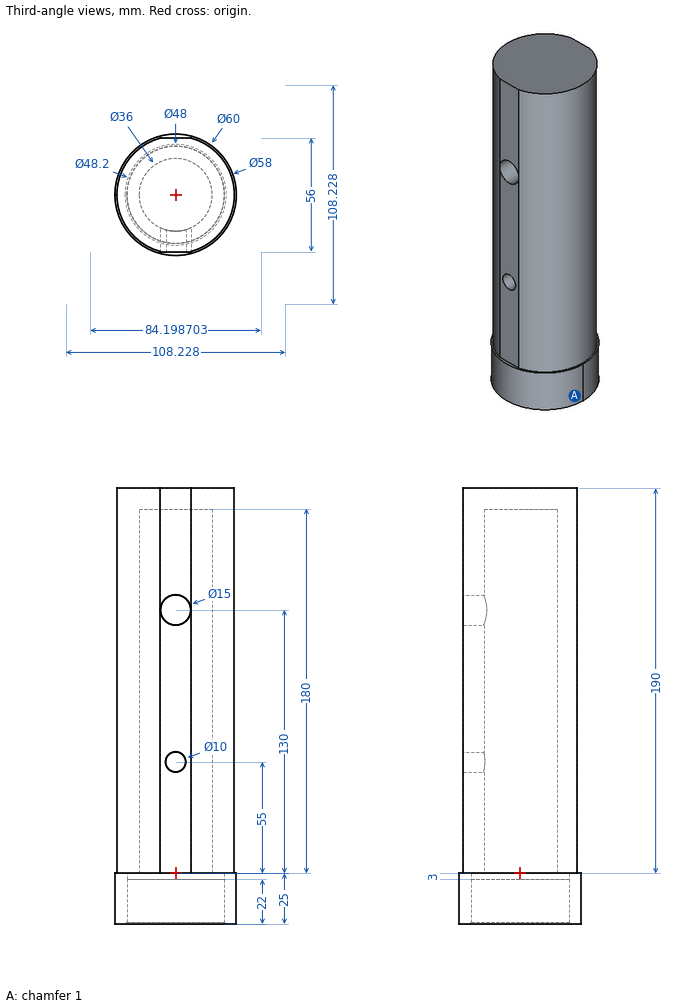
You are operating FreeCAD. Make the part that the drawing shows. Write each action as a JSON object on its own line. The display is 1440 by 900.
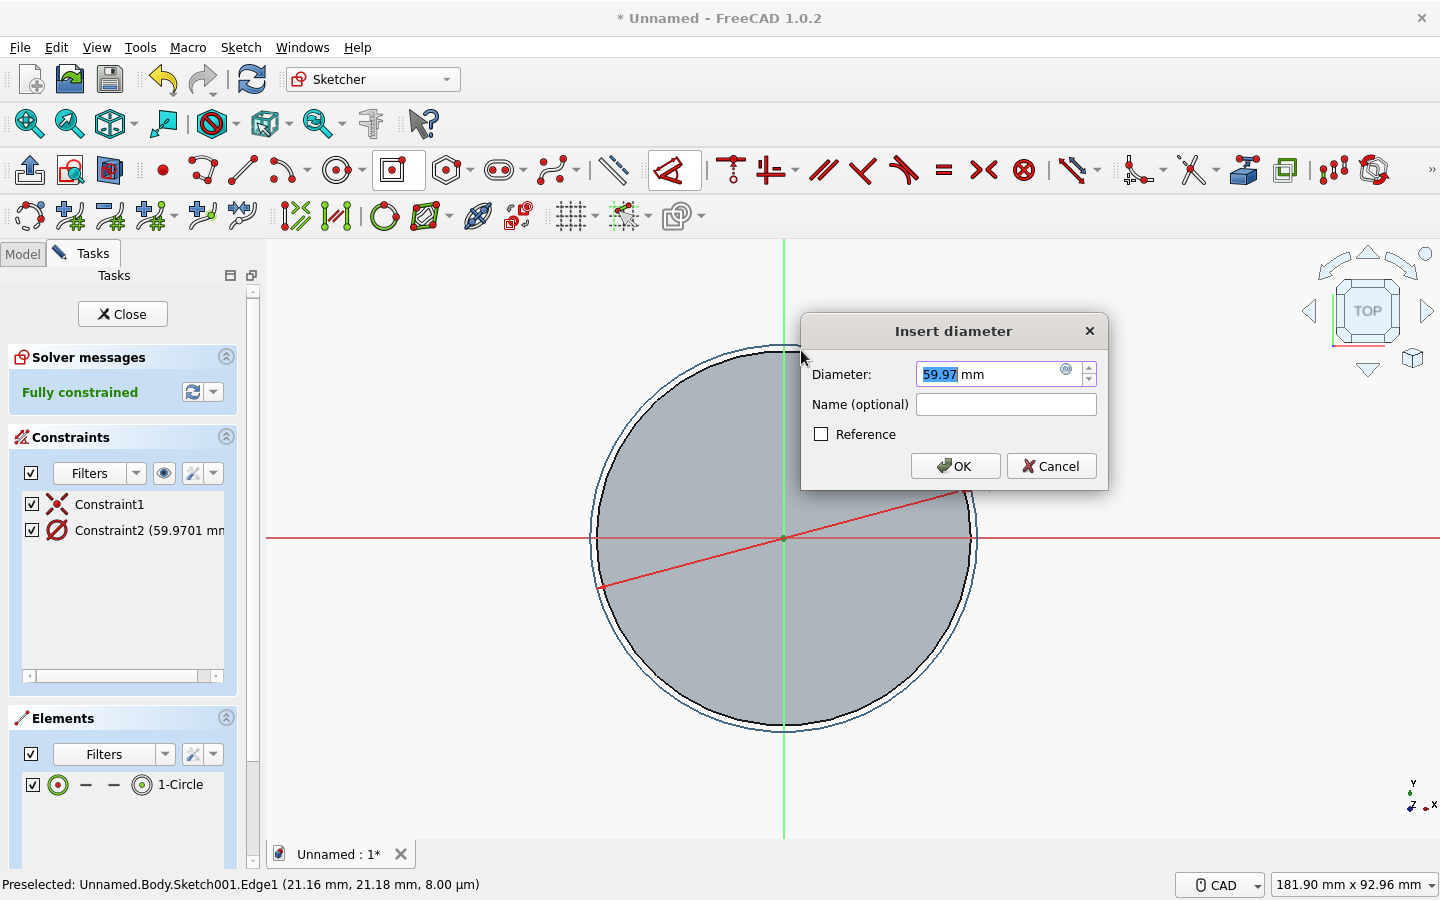
{"action": "type", "text": "60"}
{"action": "key", "text": "Return"}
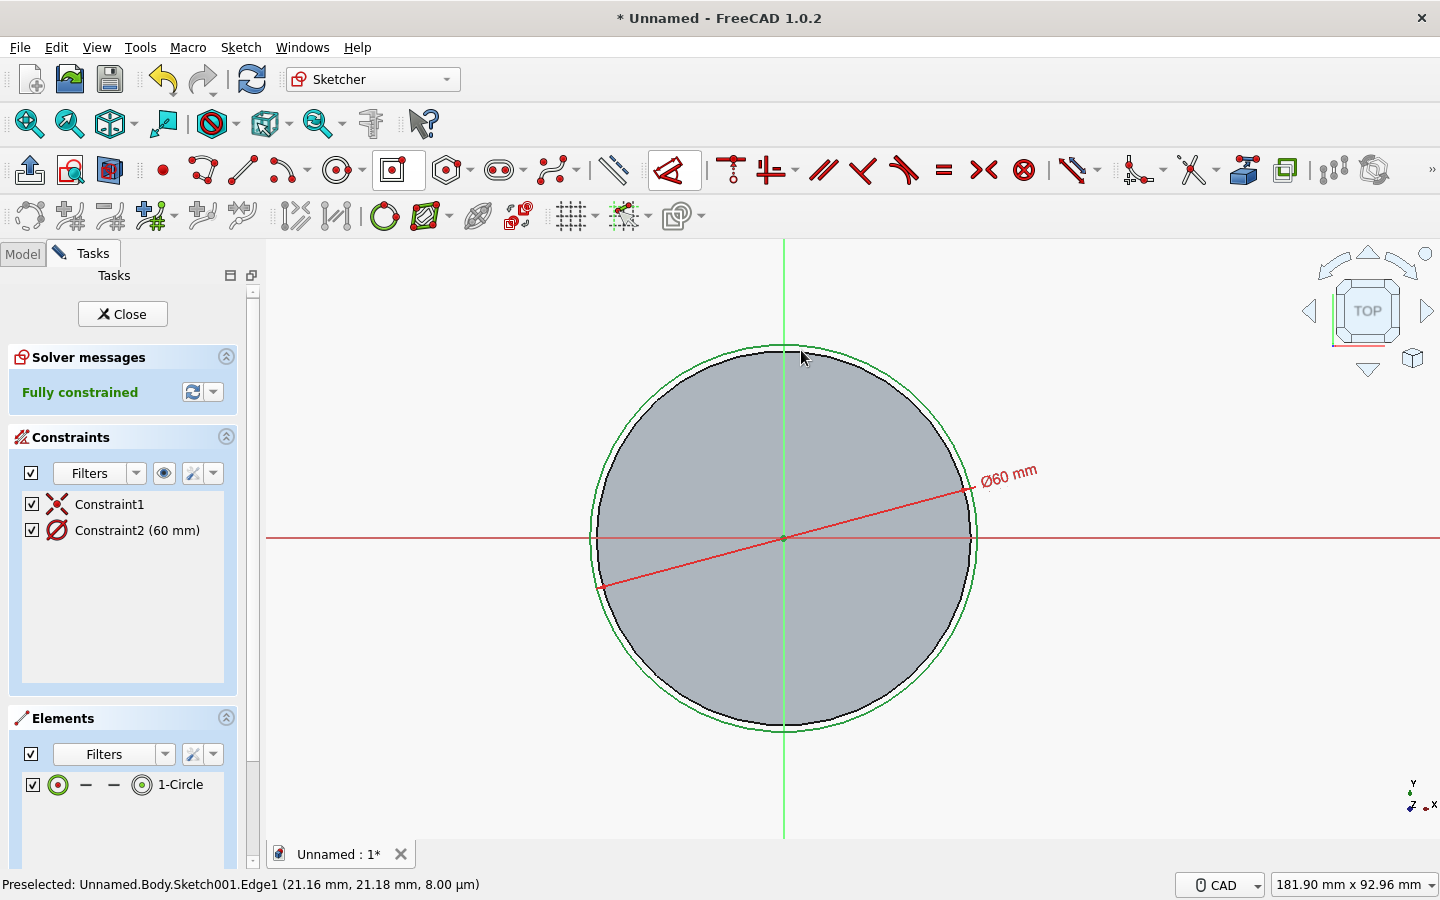
{"action": "left_click", "coordinate": [123, 314]}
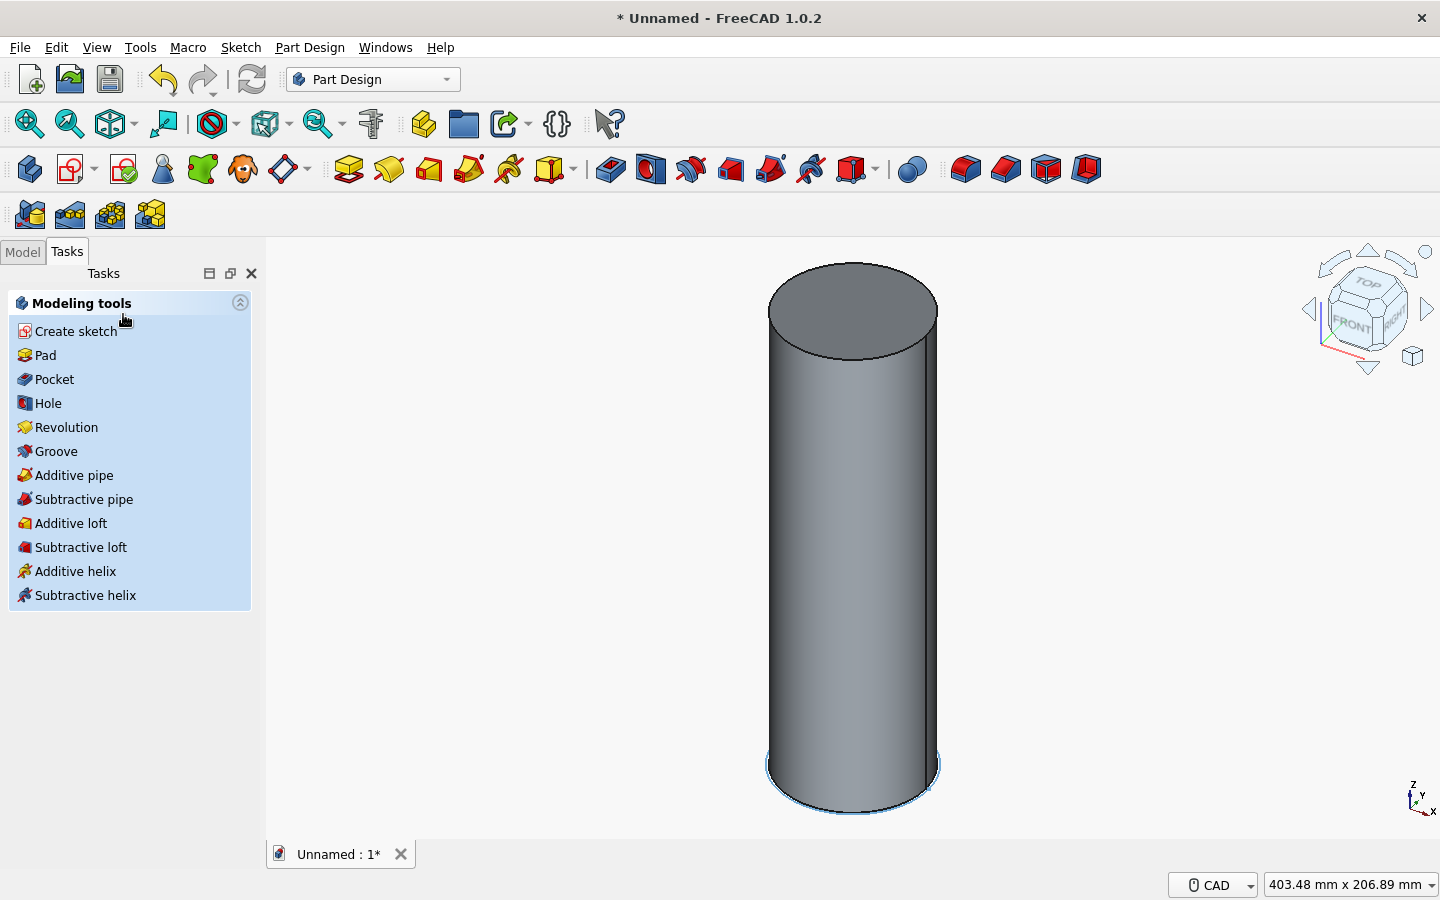
{"action": "left_click", "coordinate": [350, 170]}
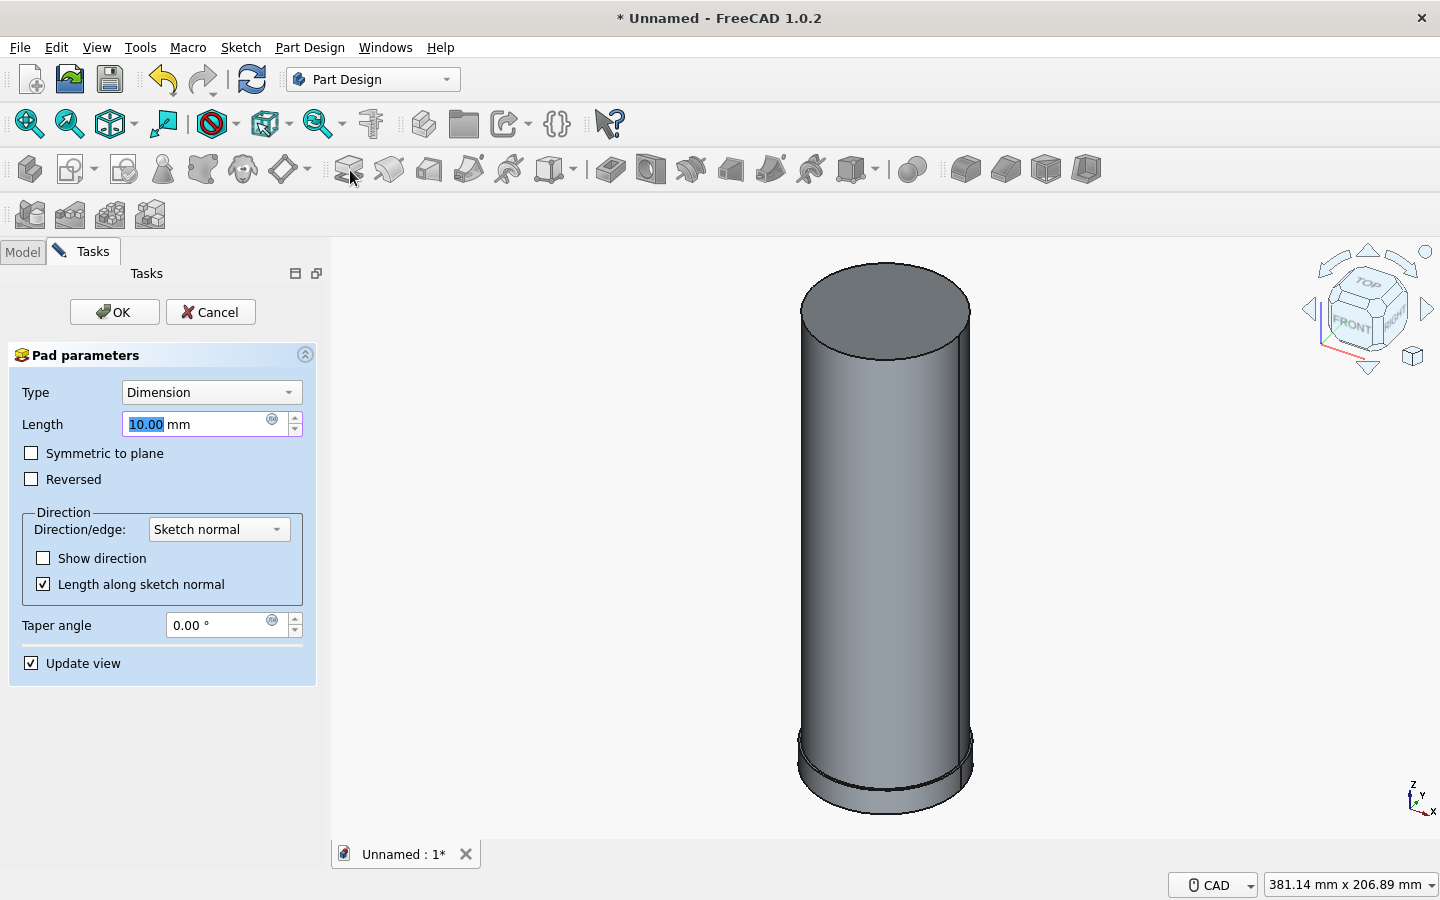
{"action": "type", "text": "25"}
{"action": "key", "text": "Tab"}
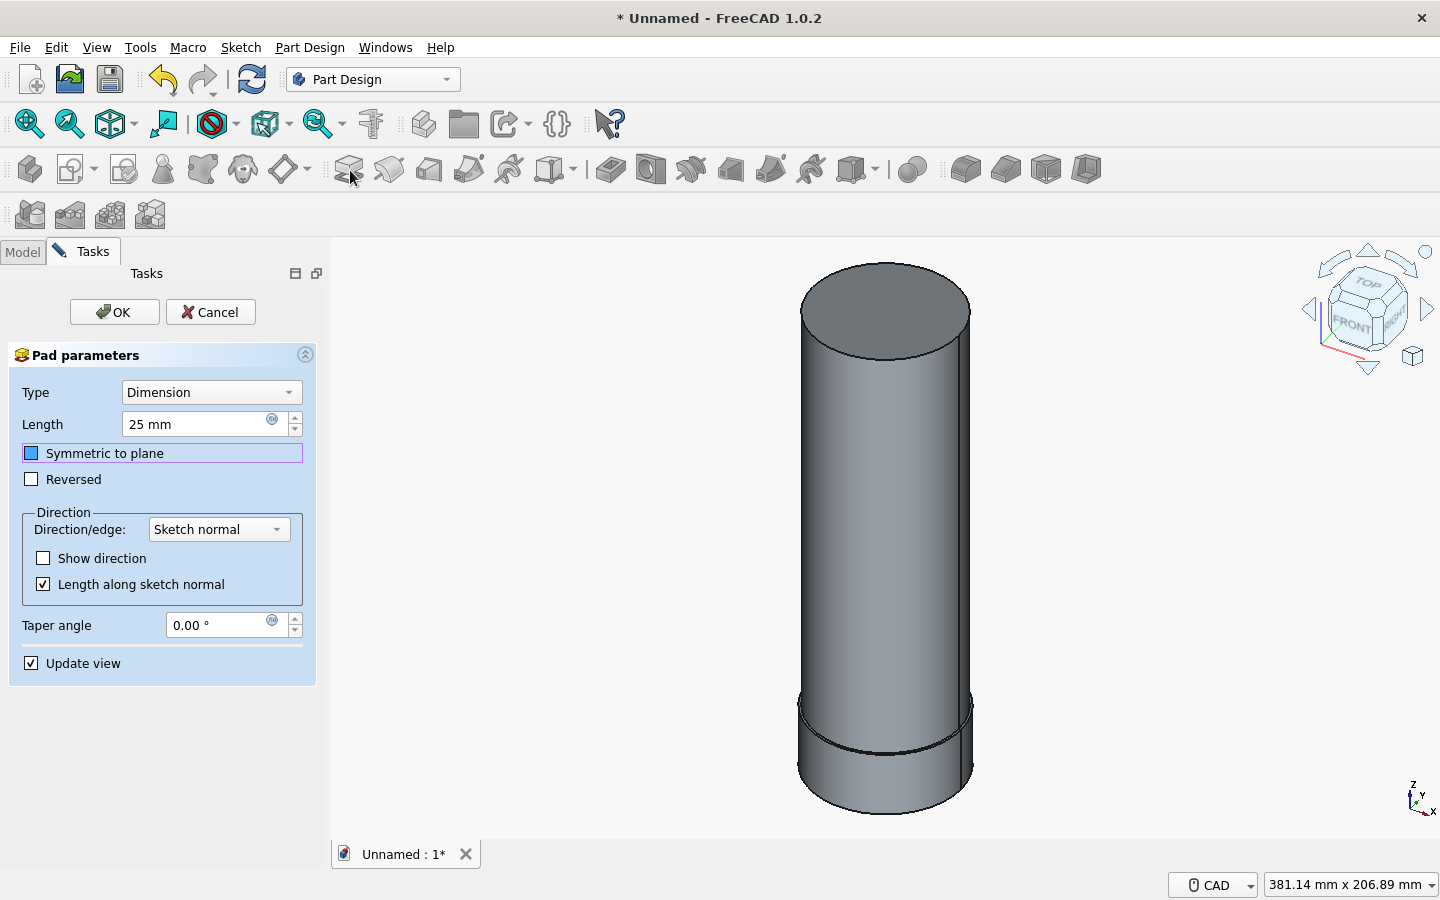
{"action": "left_click", "coordinate": [30, 479]}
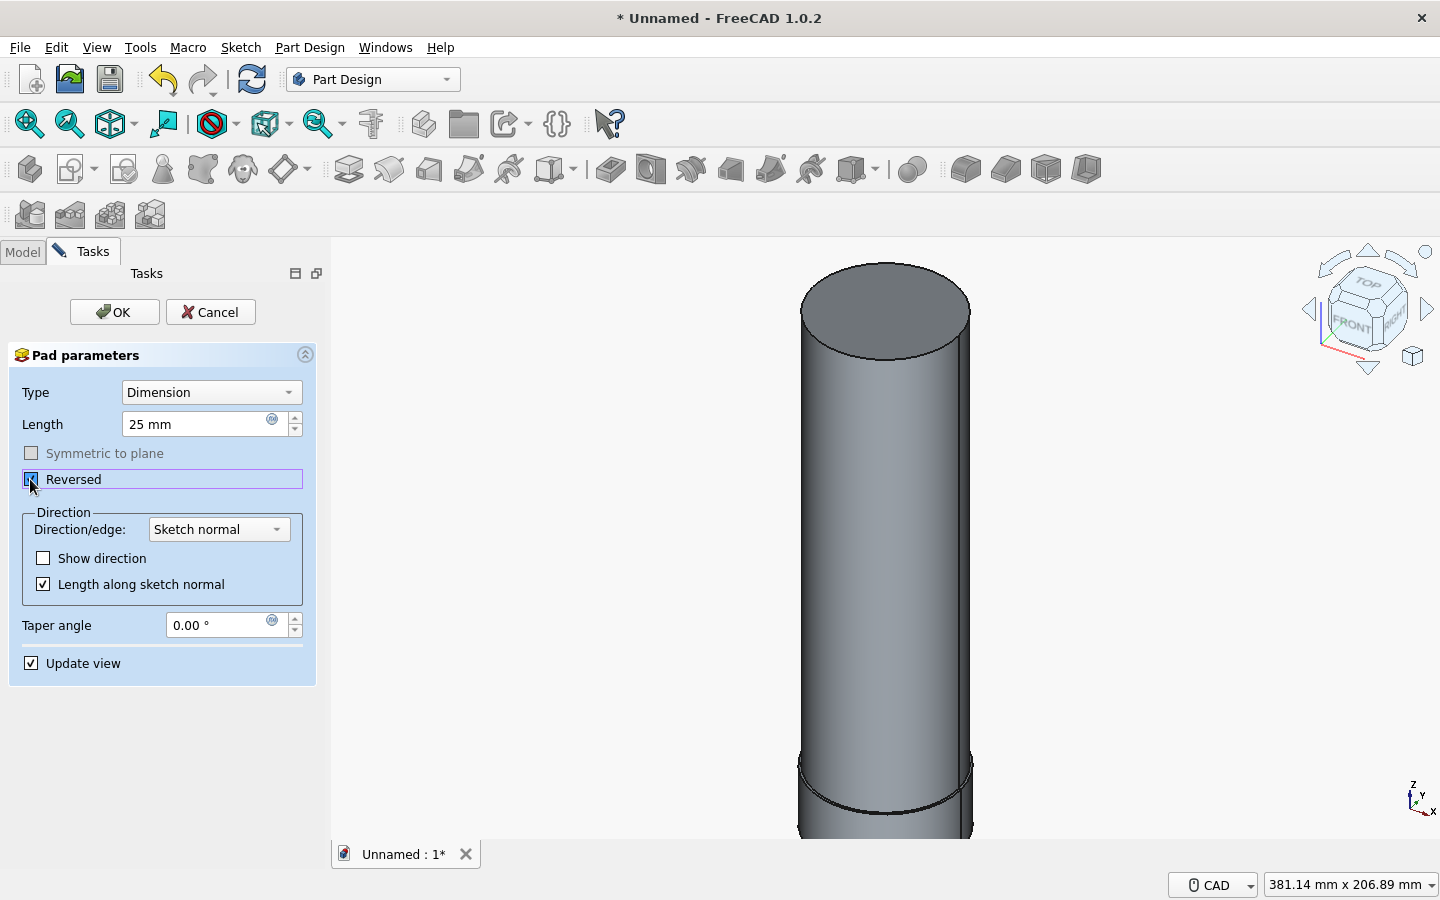
{"action": "left_click", "coordinate": [115, 312]}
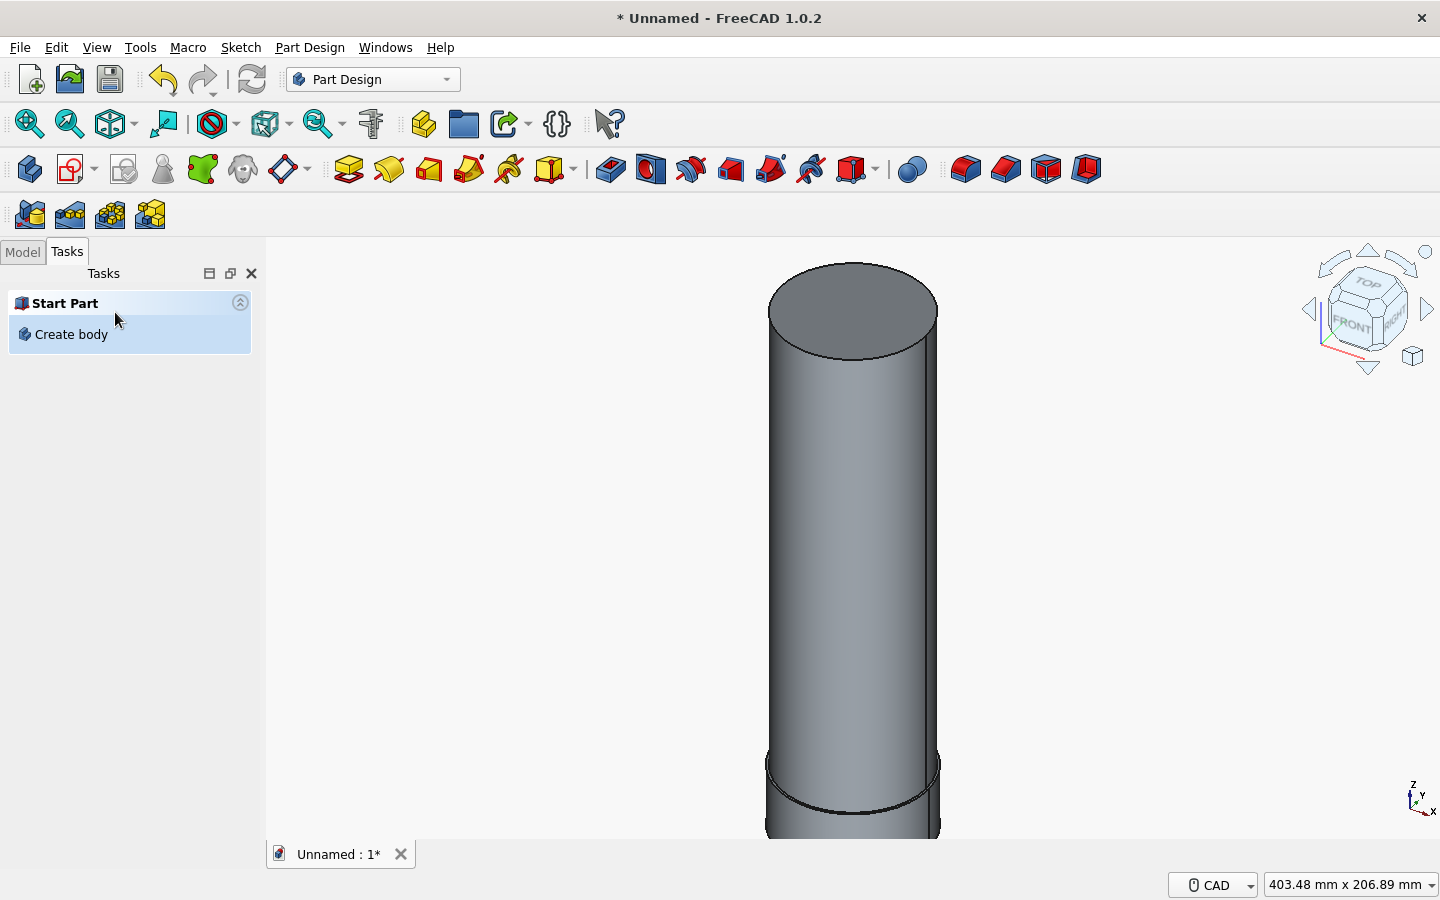
{"action": "left_click", "coordinate": [30, 124]}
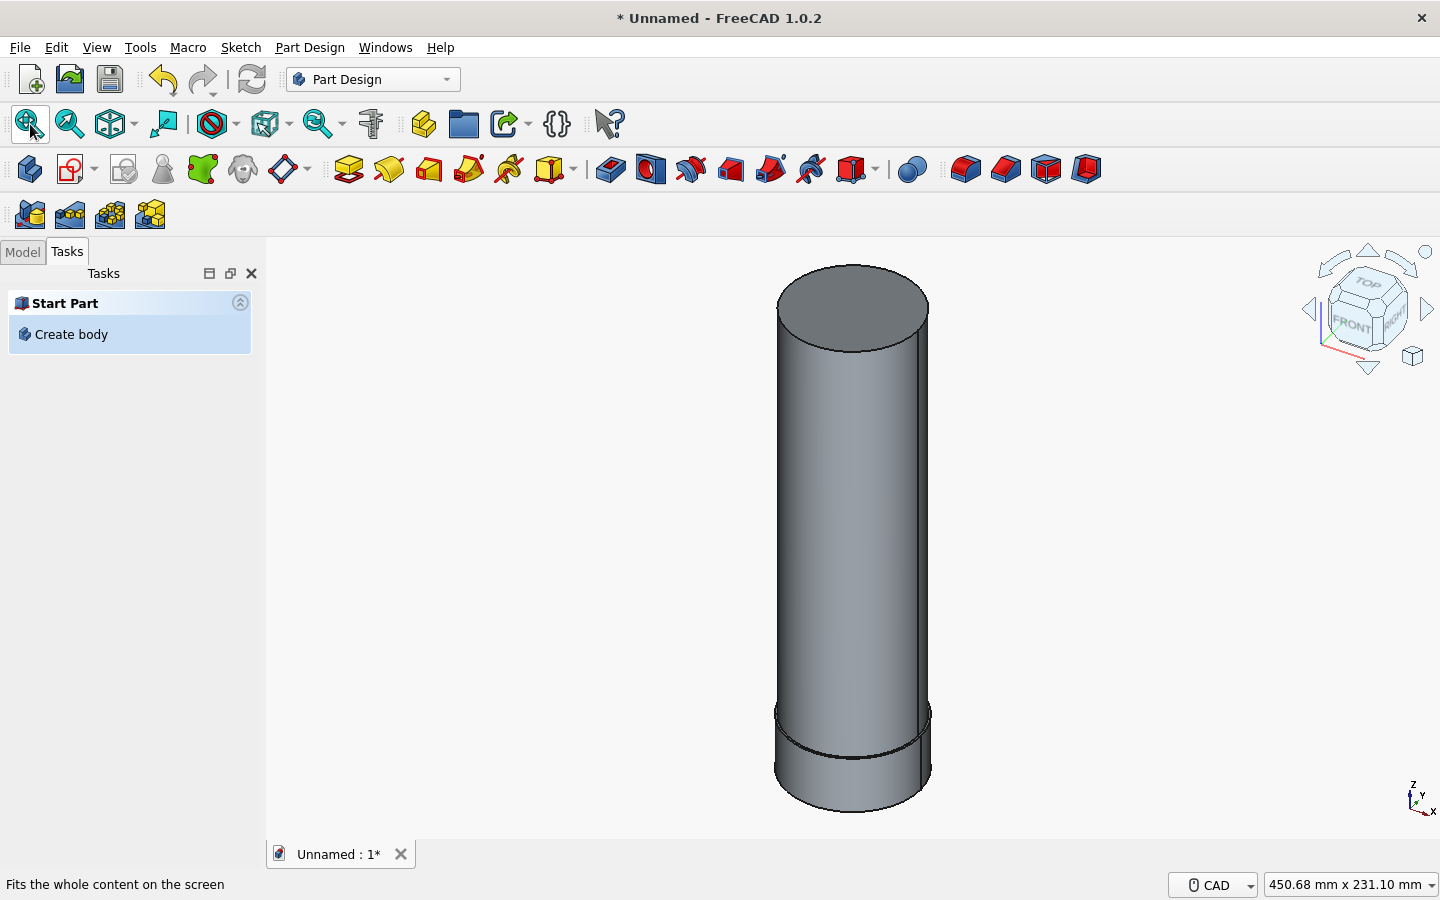
{"action": "left_click", "coordinate": [853, 308]}